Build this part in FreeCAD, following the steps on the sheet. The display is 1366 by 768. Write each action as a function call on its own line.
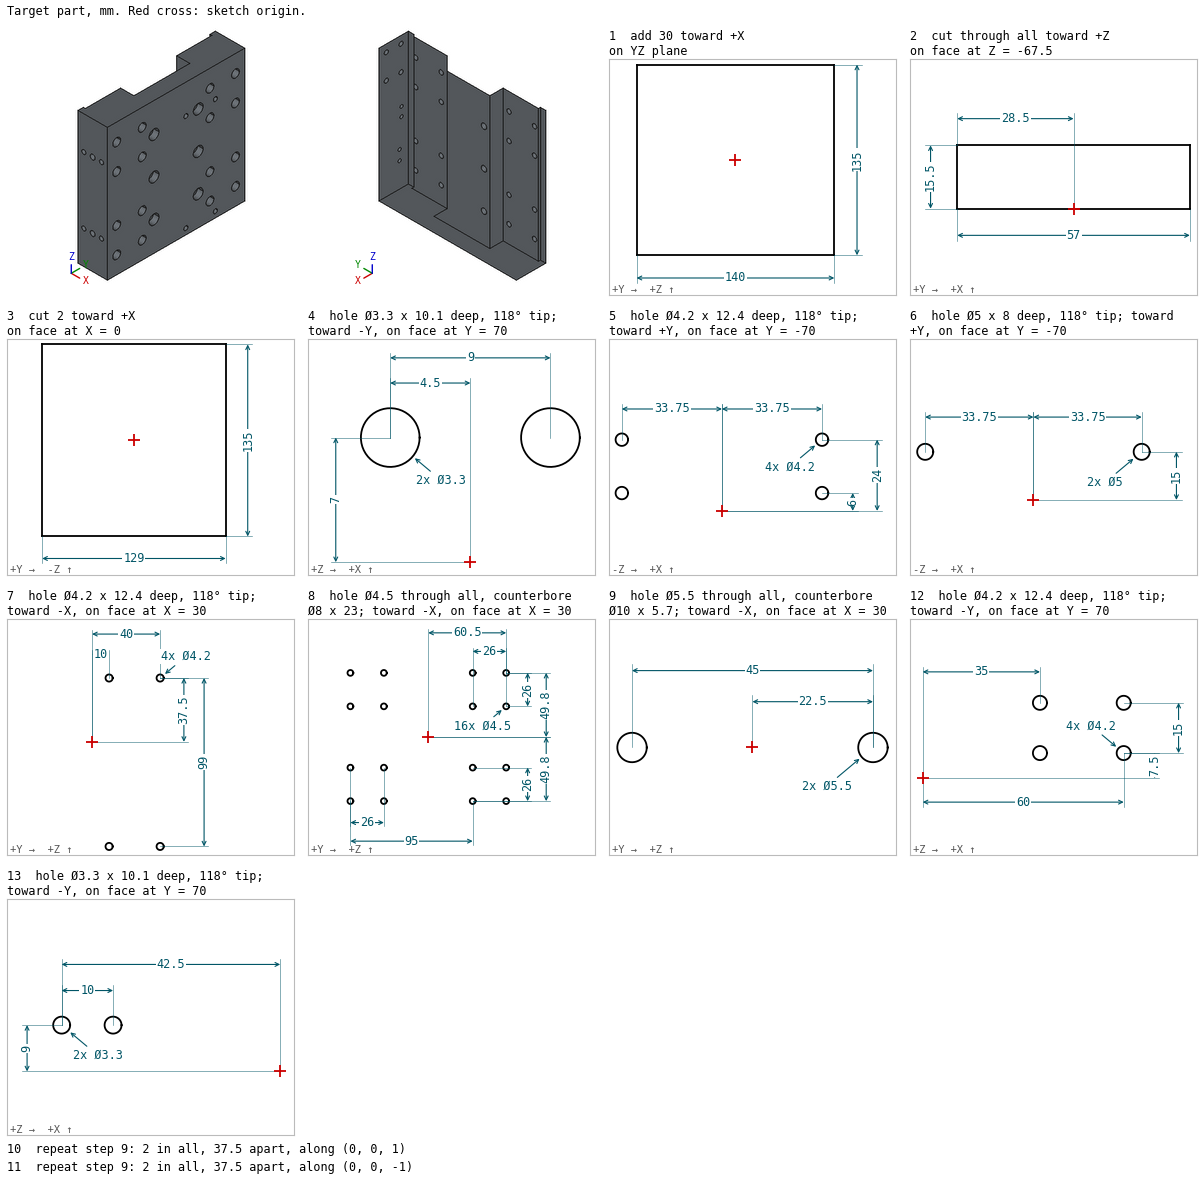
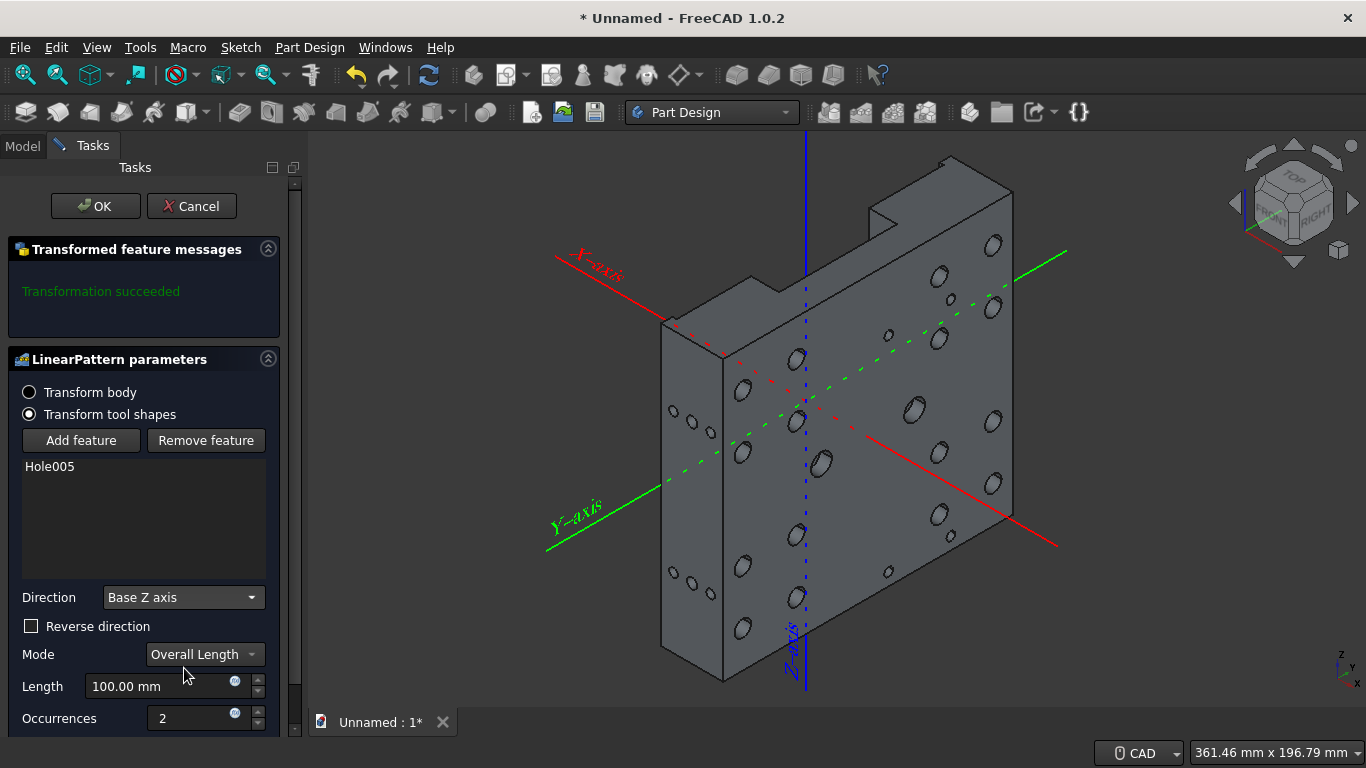
click(206, 654)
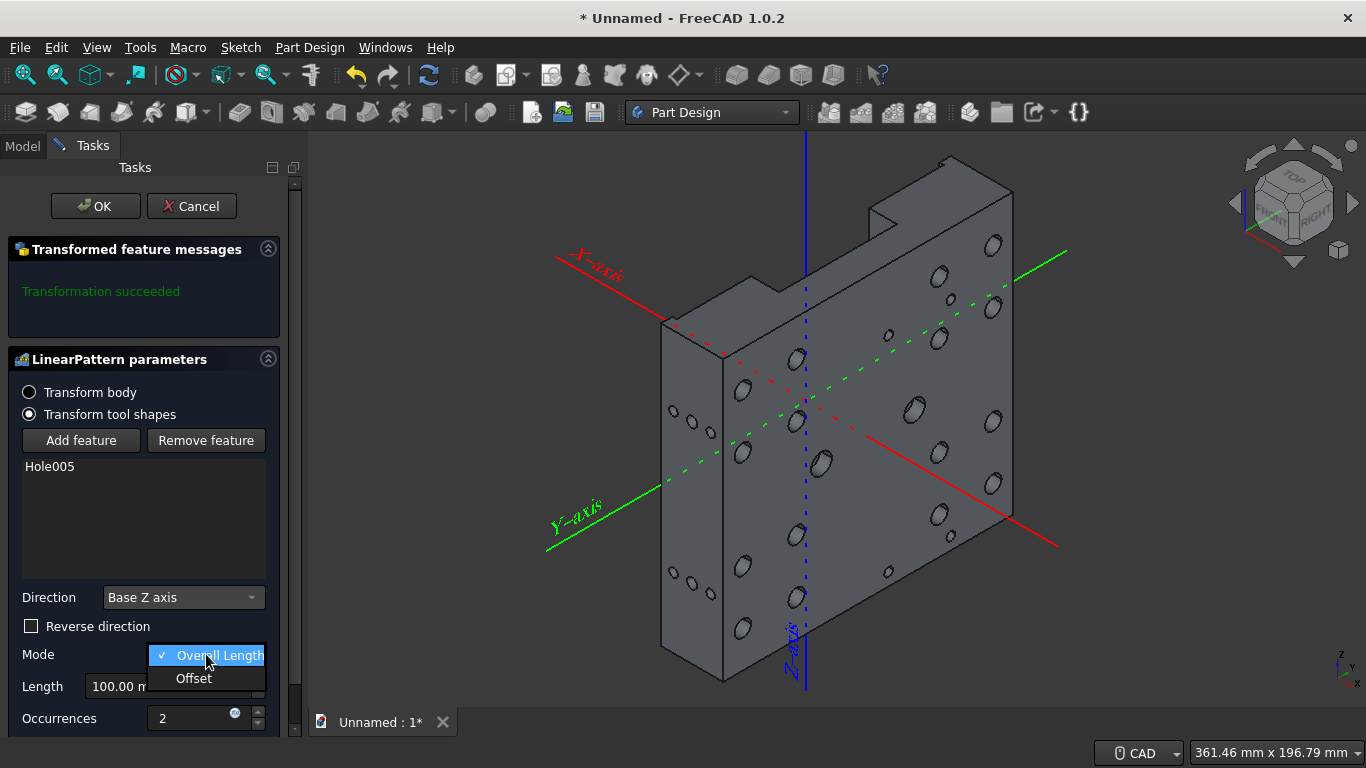
click(206, 678)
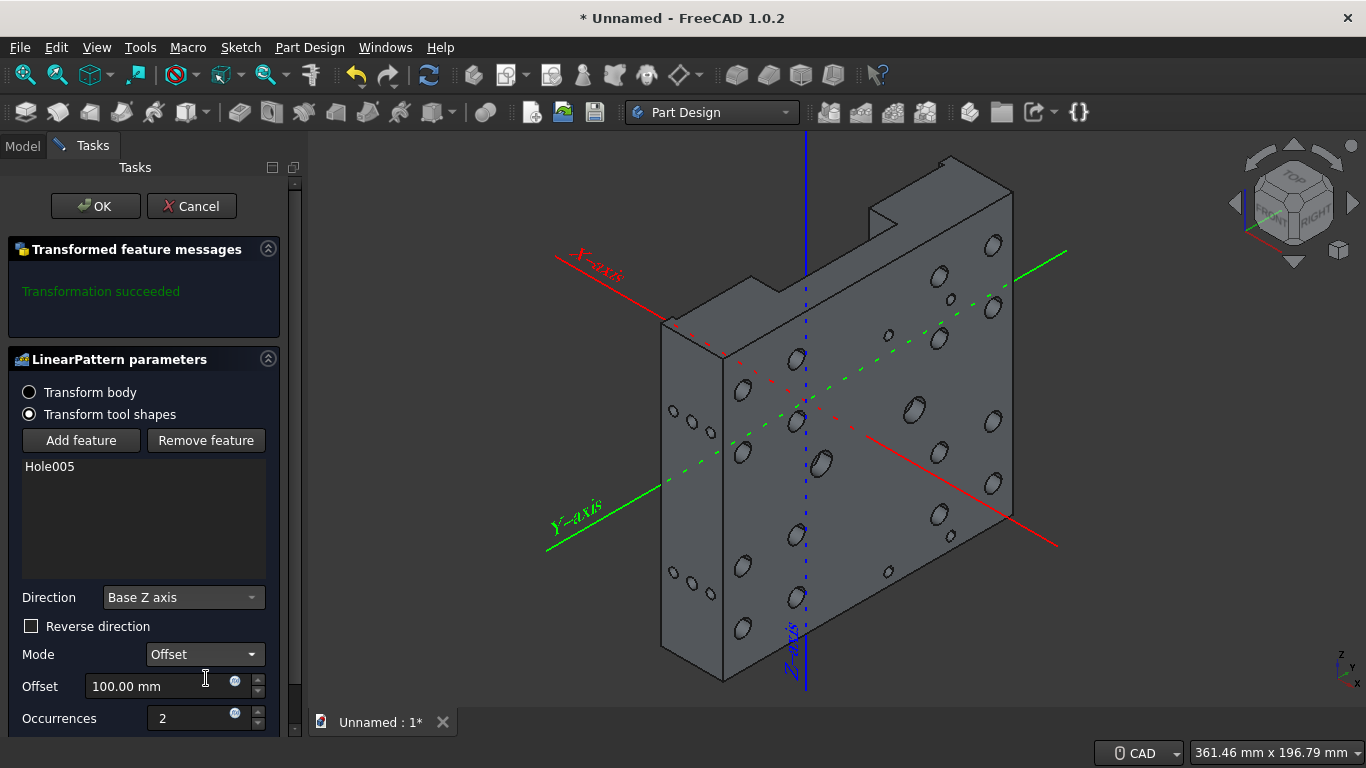
triple_click(168, 686)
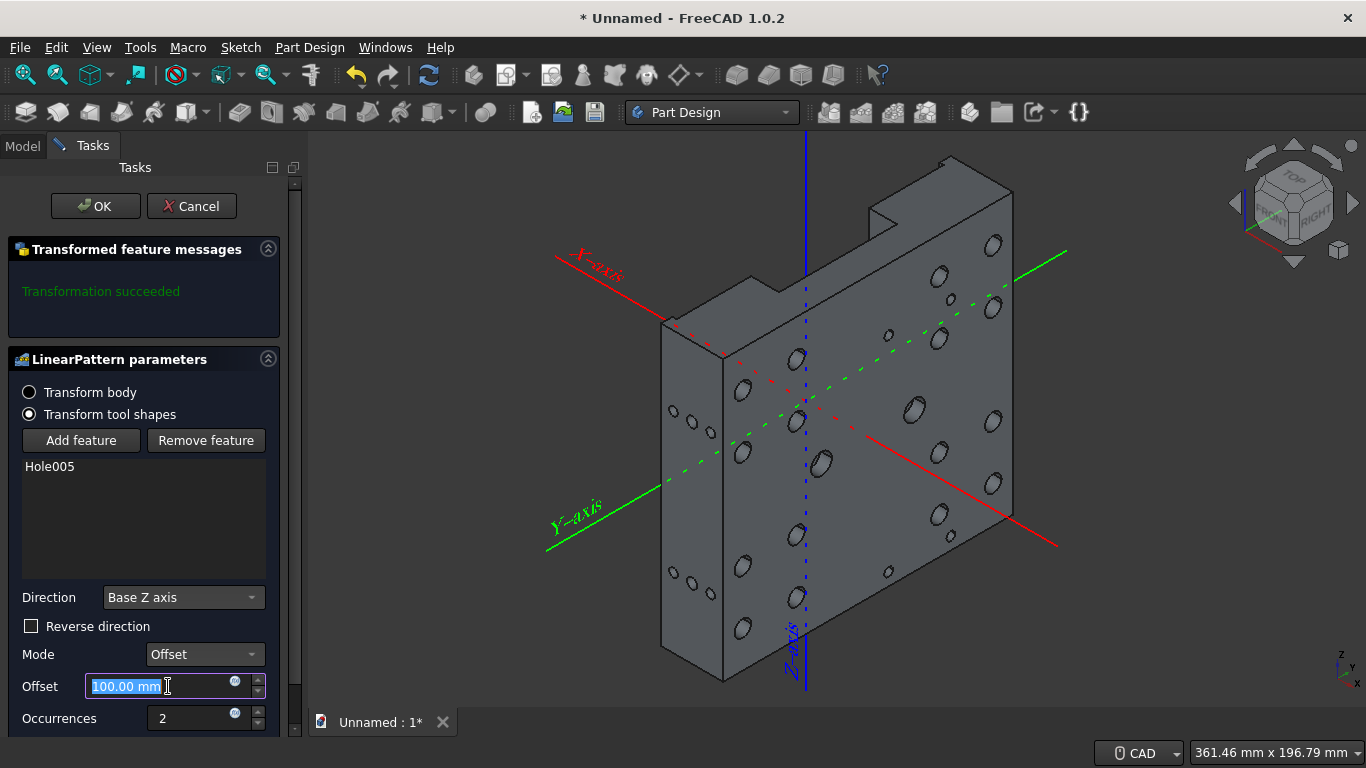
text(37.5)
key(Tab)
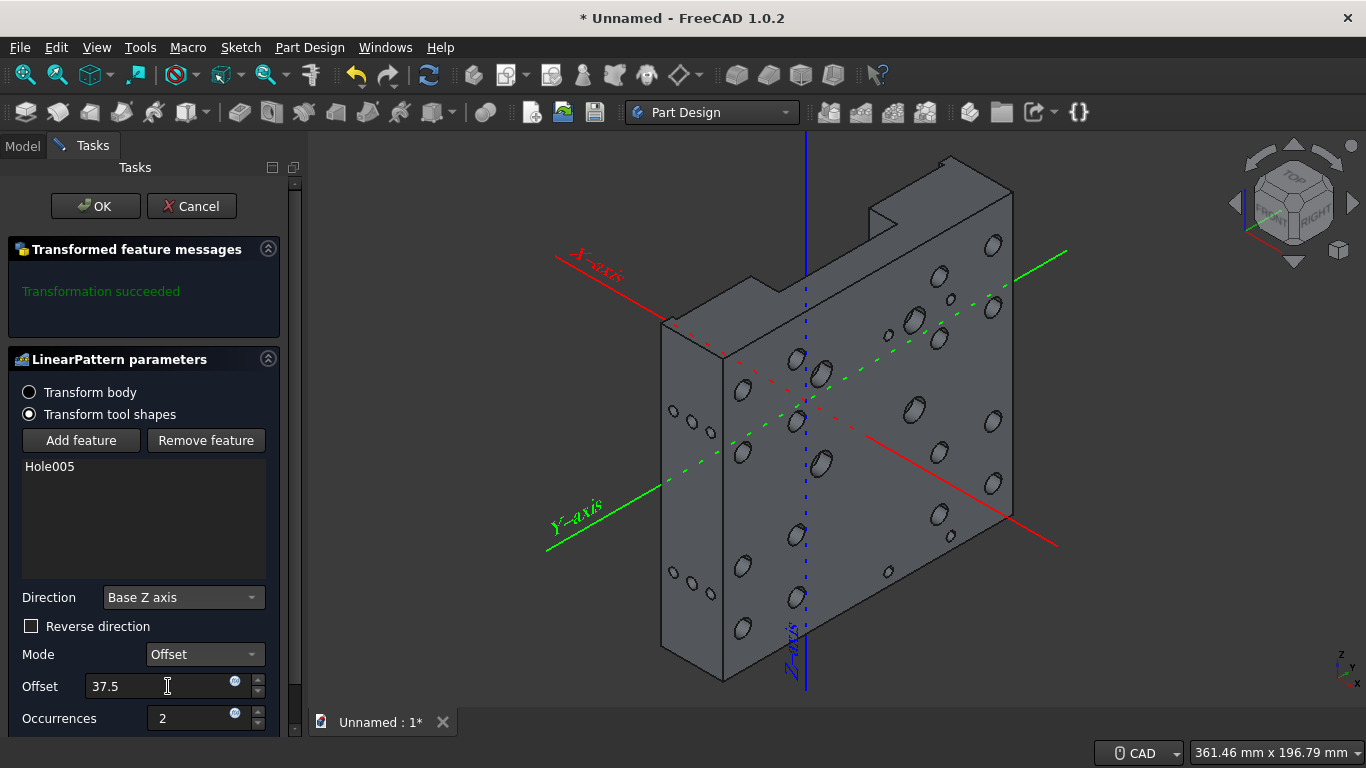
triple_click(198, 718)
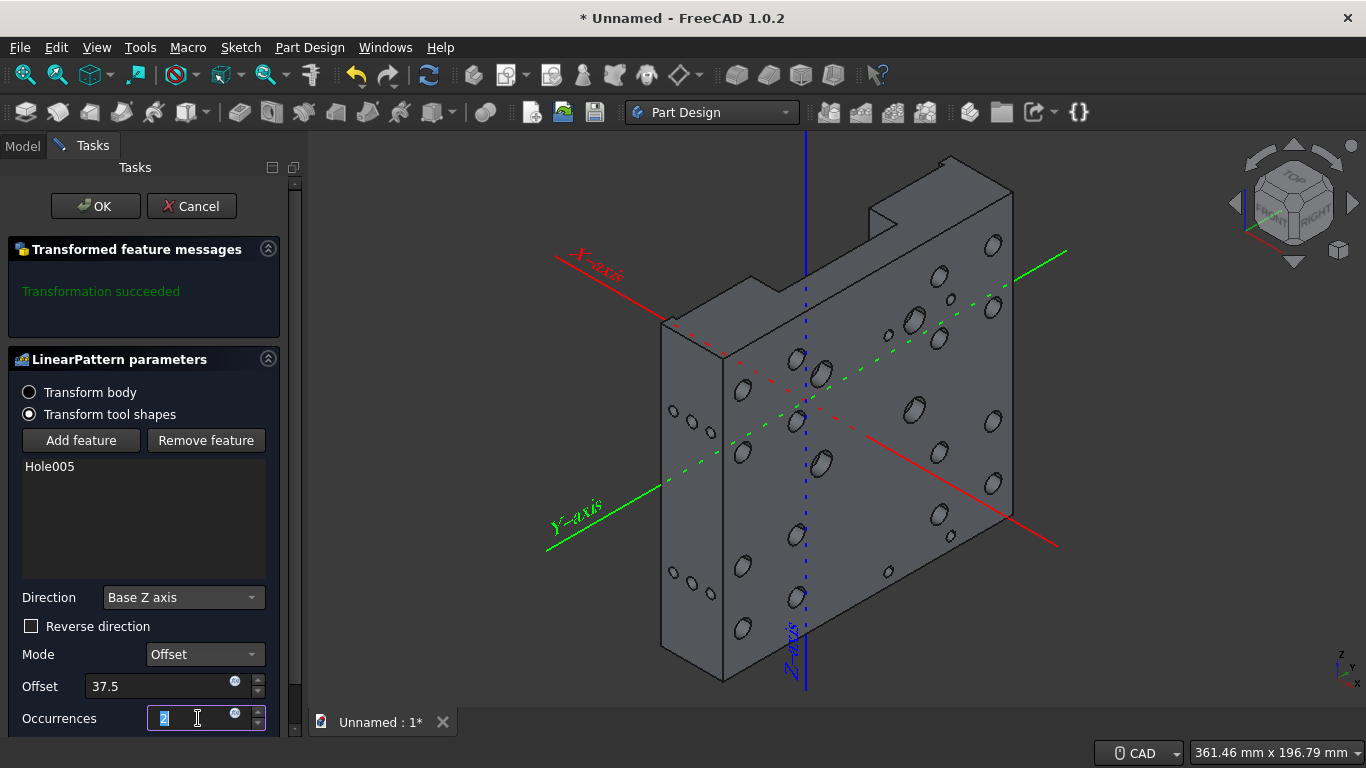
text(2)
key(Tab)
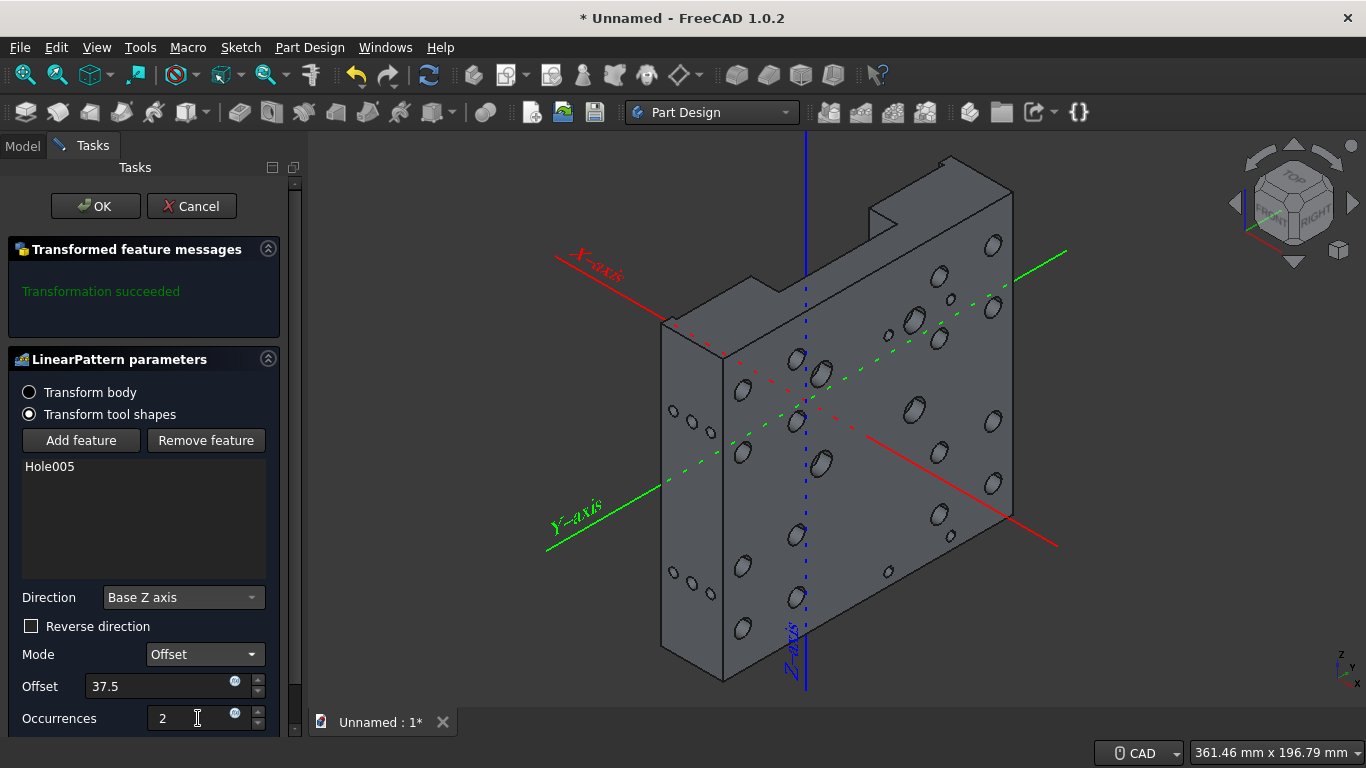
click(96, 206)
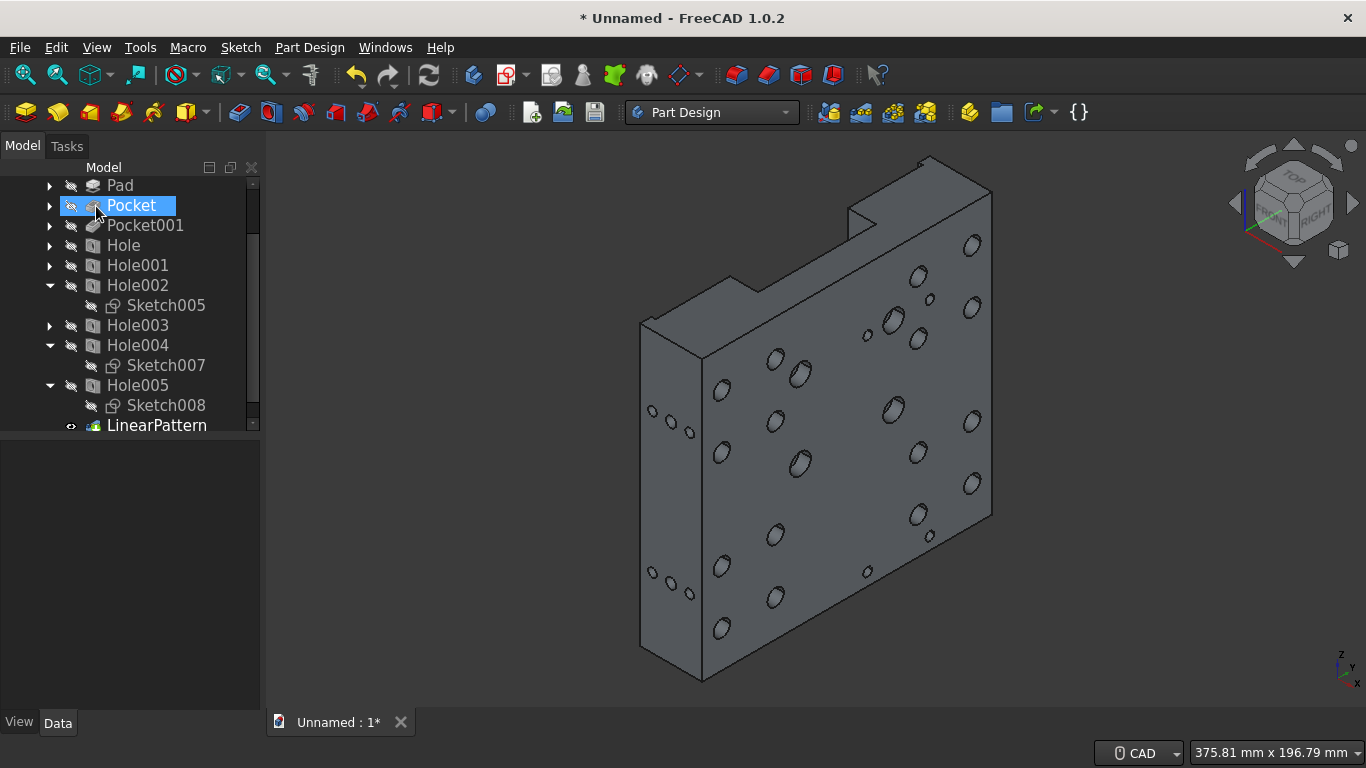
click(116, 386)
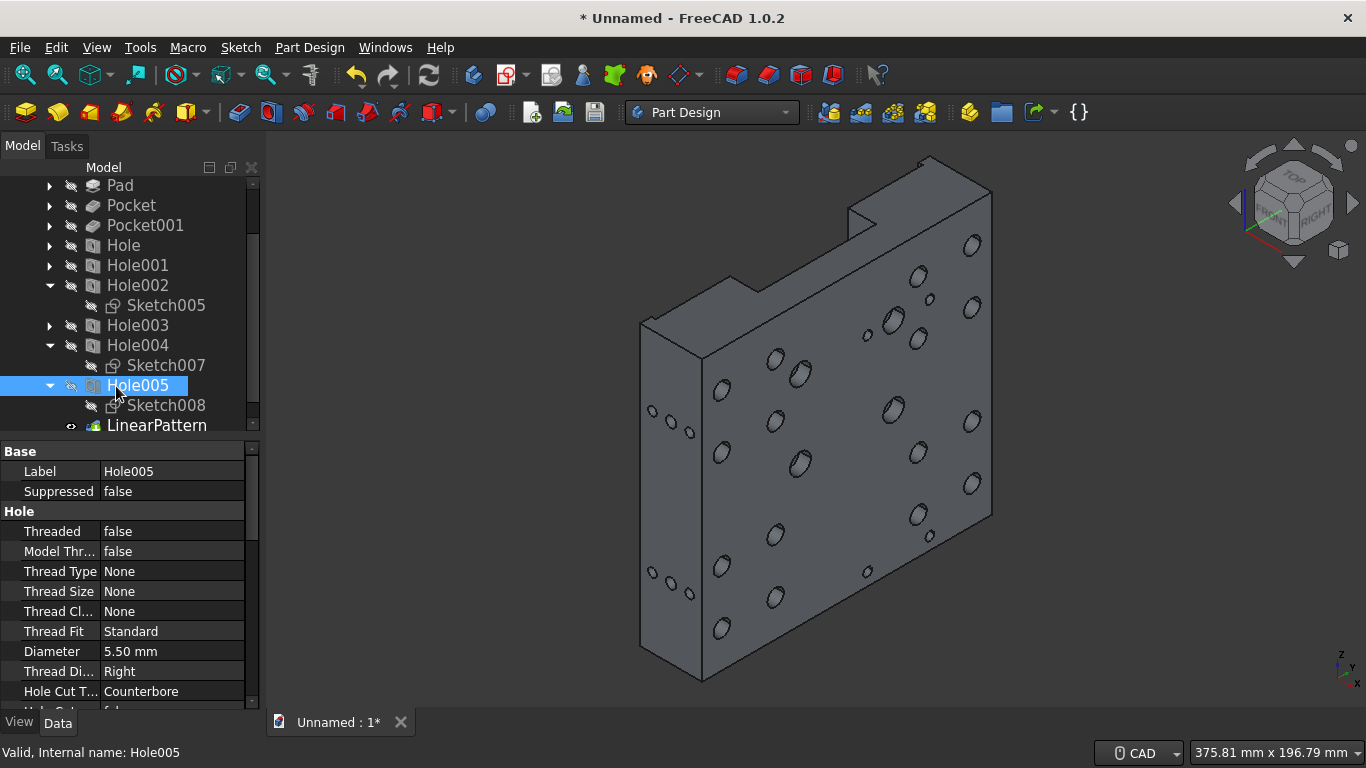
click(862, 112)